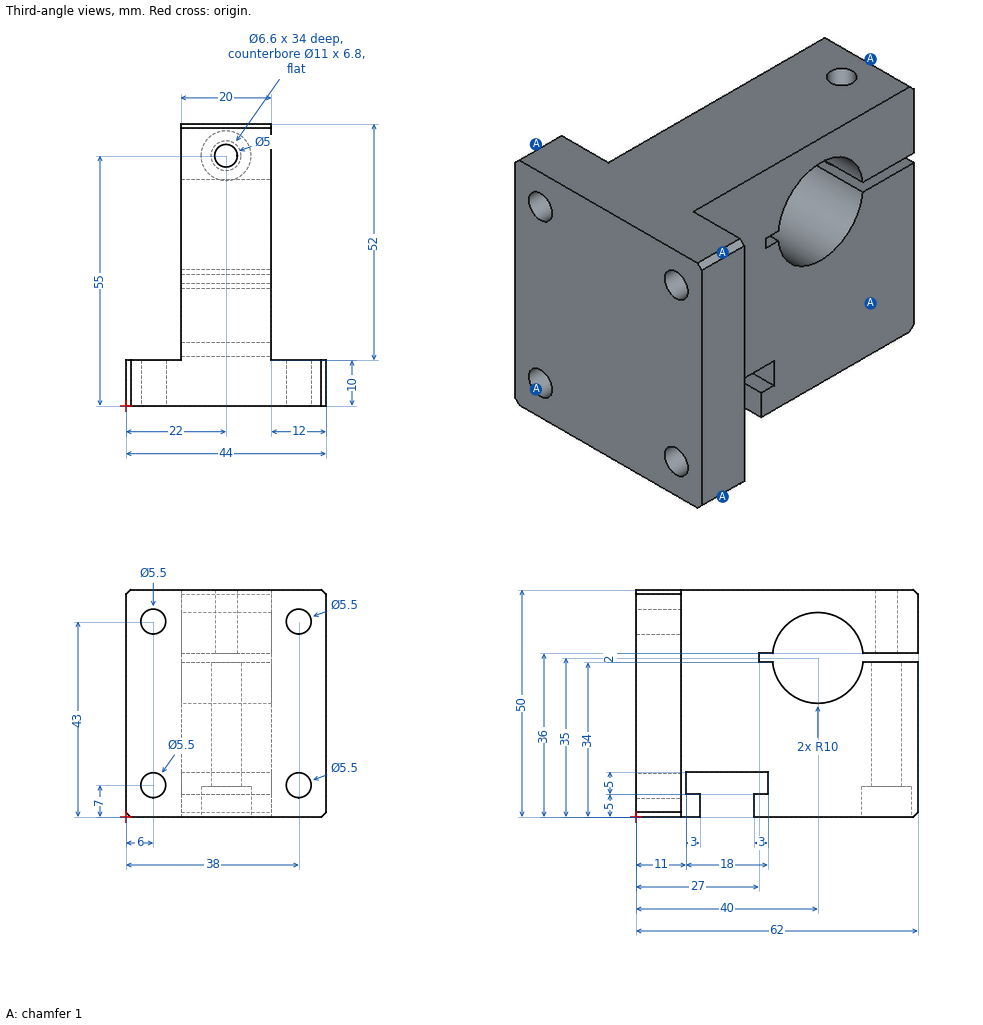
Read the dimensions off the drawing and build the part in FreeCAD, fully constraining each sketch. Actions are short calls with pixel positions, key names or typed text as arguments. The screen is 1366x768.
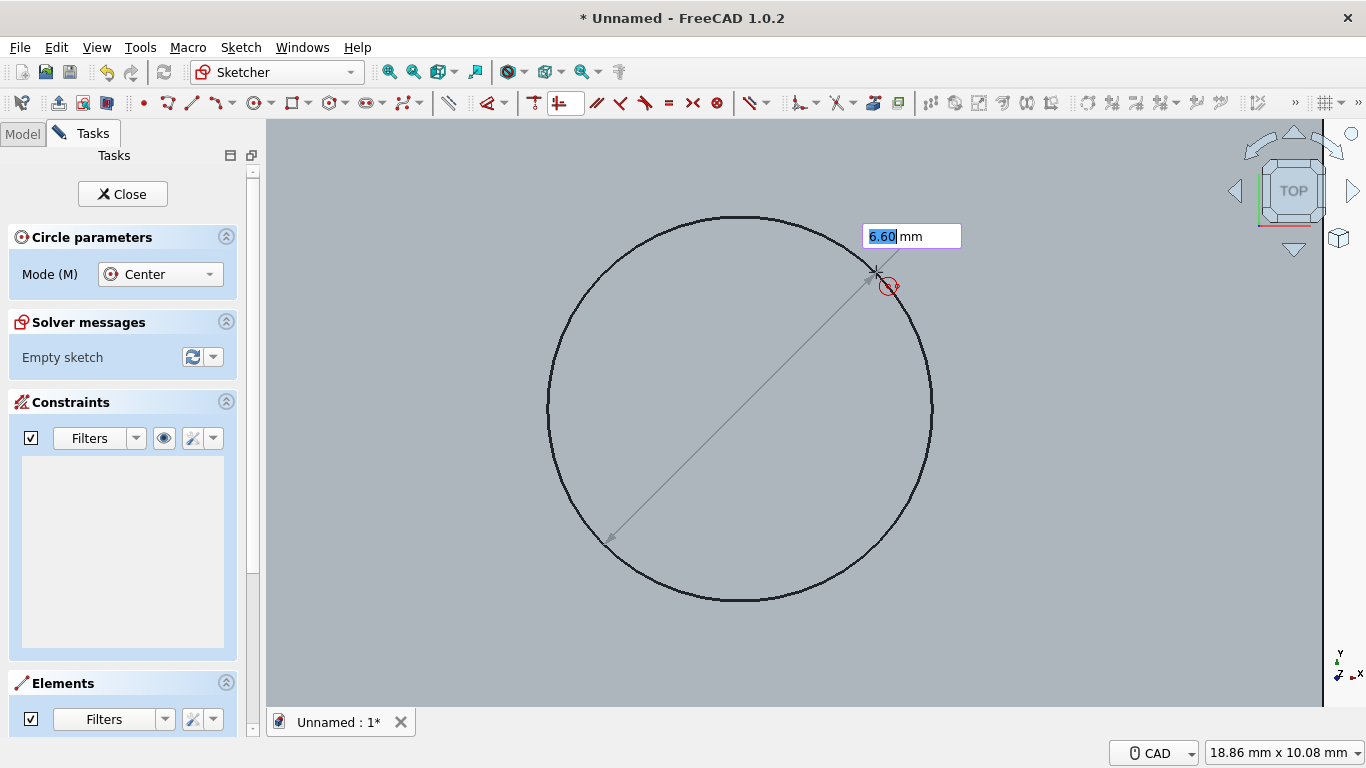
text(6.6)
key(Return)
key(Escape)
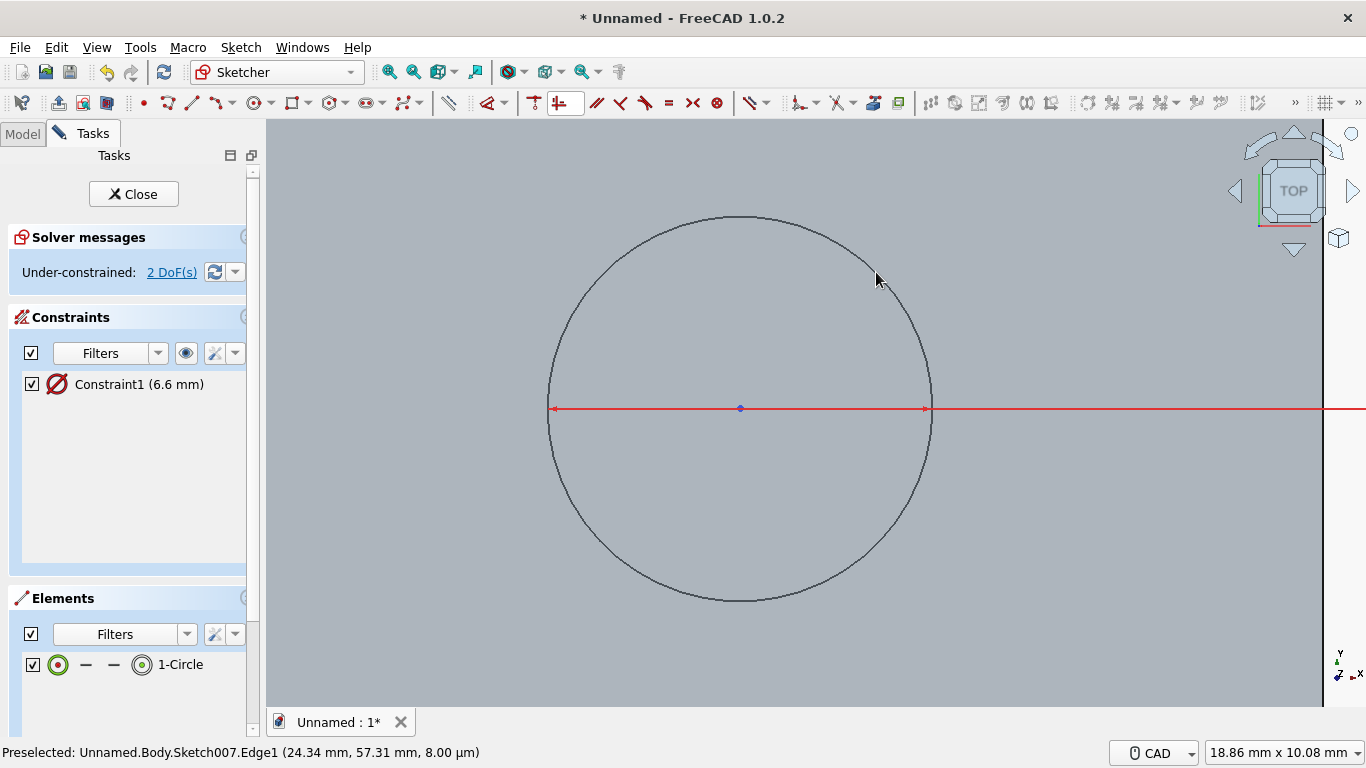
click(488, 104)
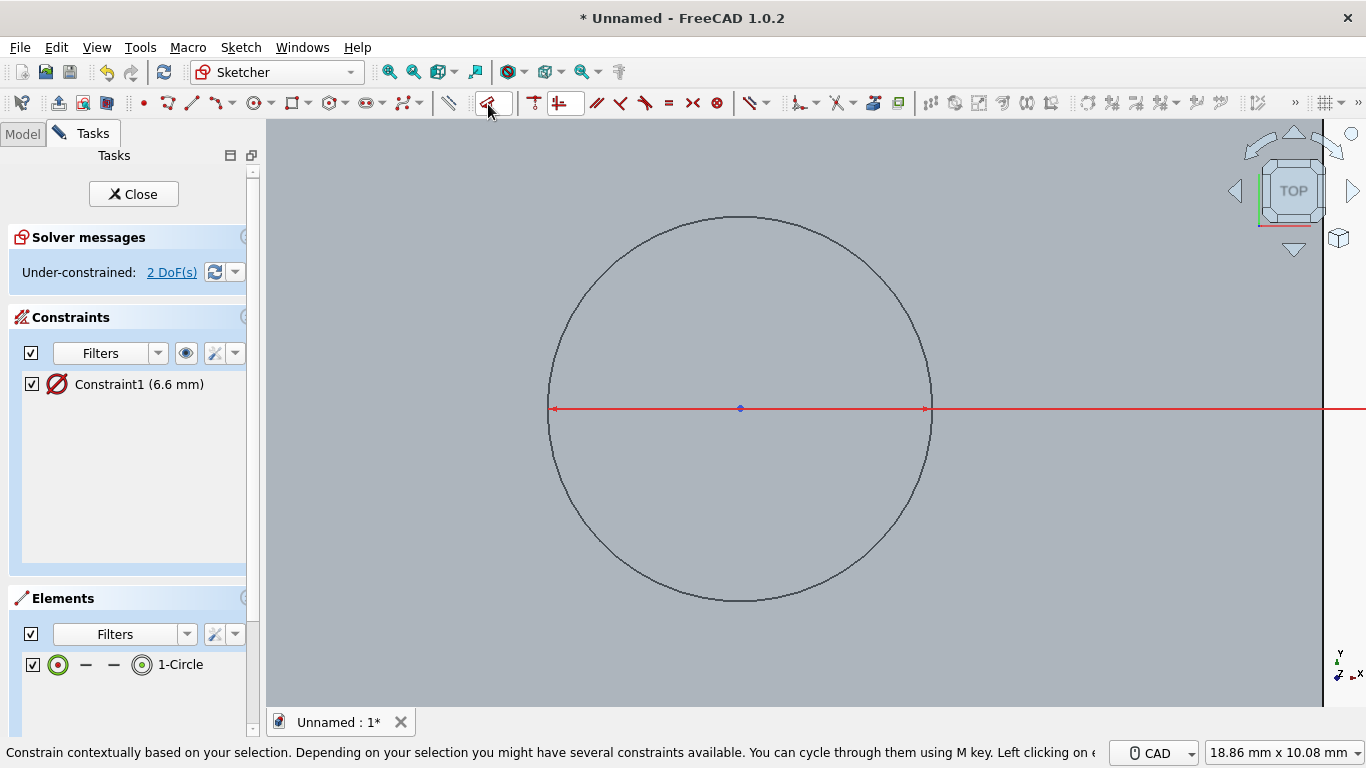
click(740, 409)
click(517, 375)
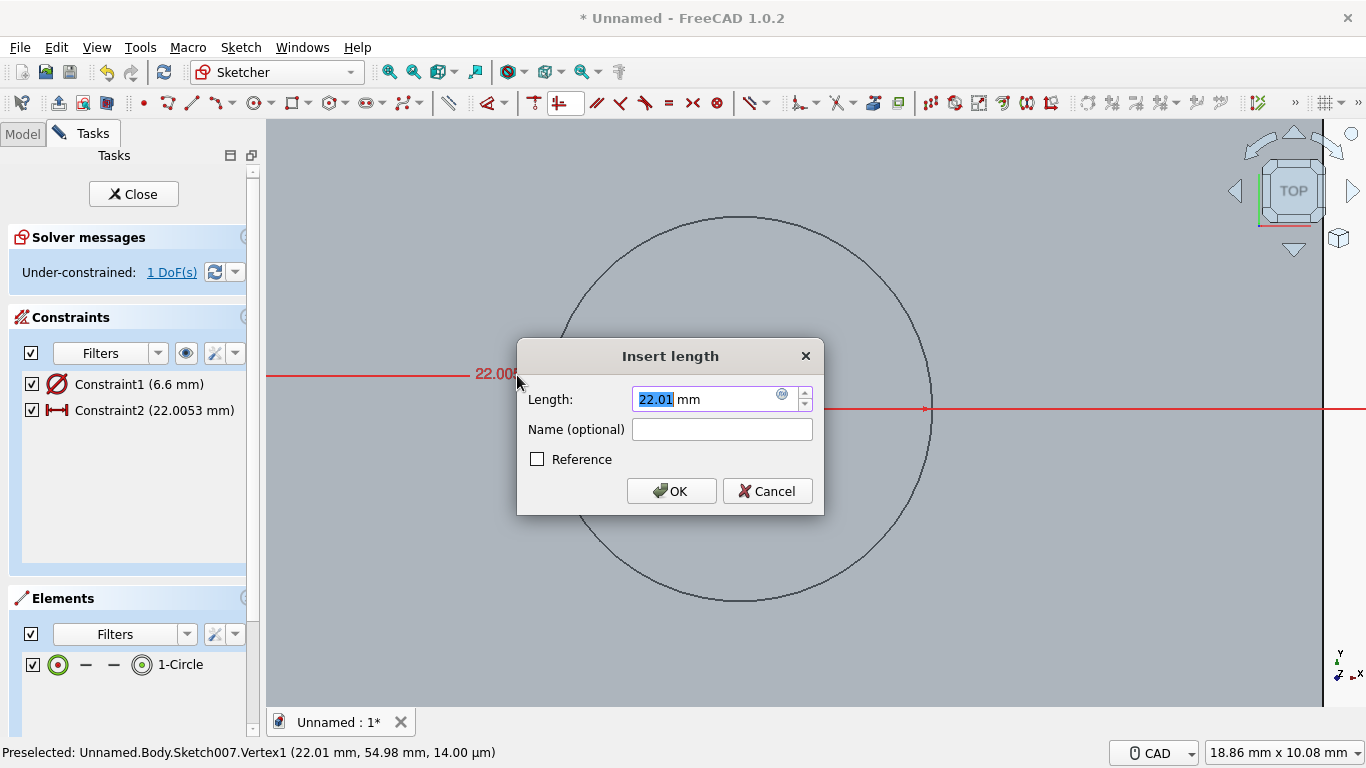
text(22)
key(Return)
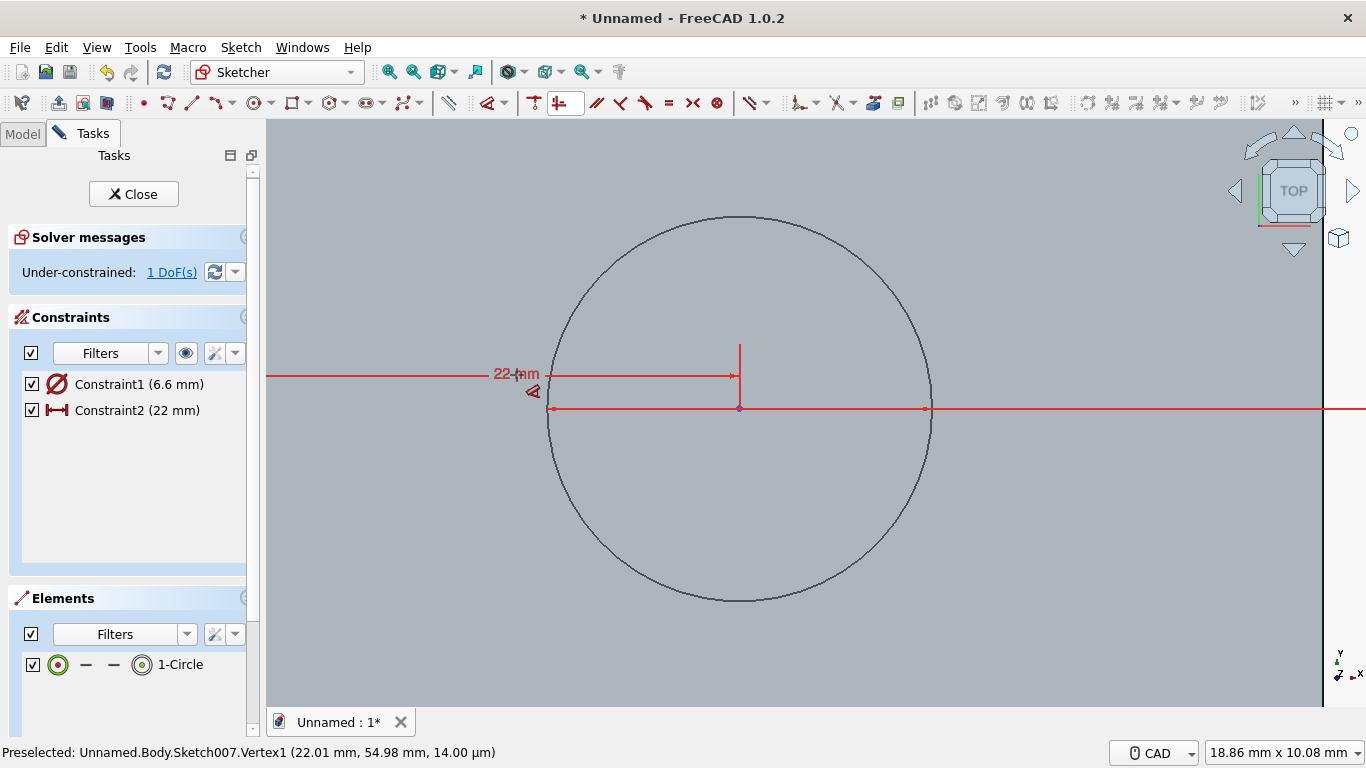
click(740, 409)
click(774, 544)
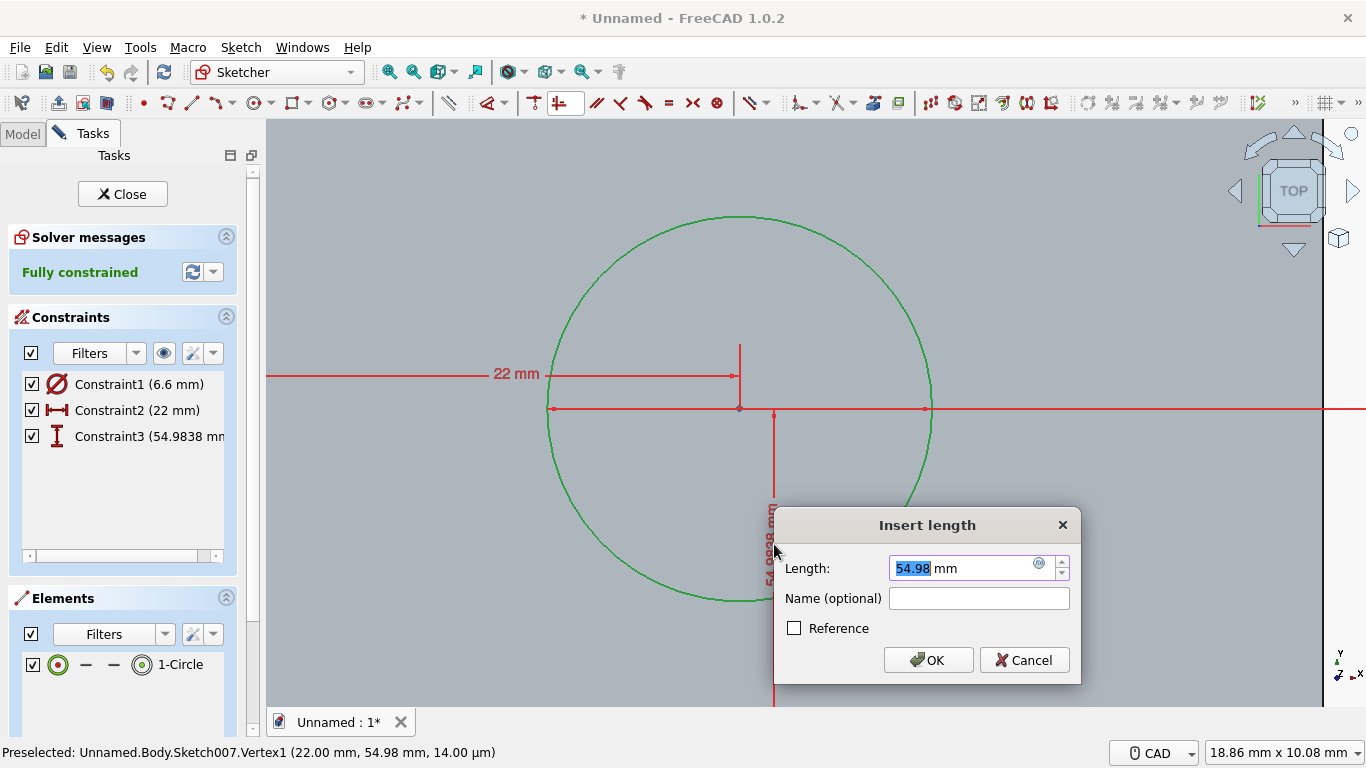
text(55)
key(Return)
key(Escape)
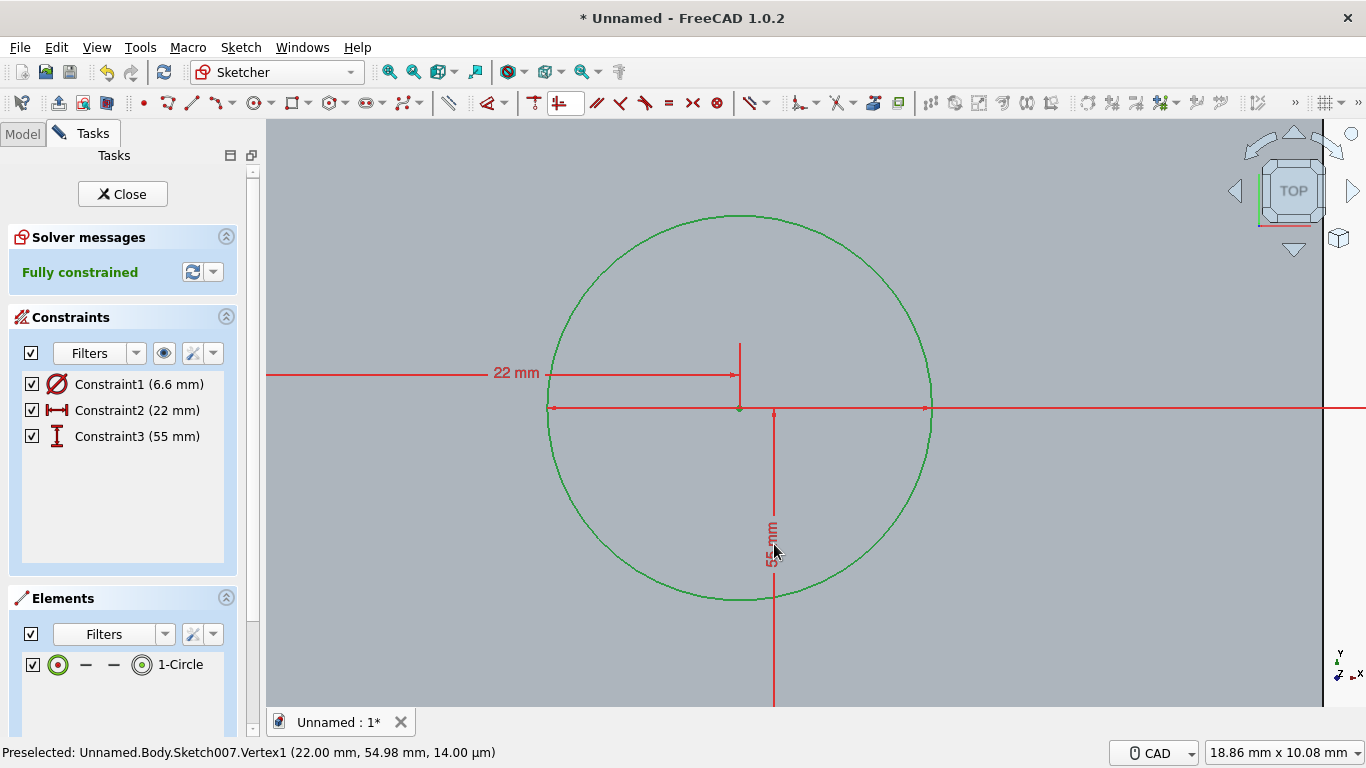
click(123, 194)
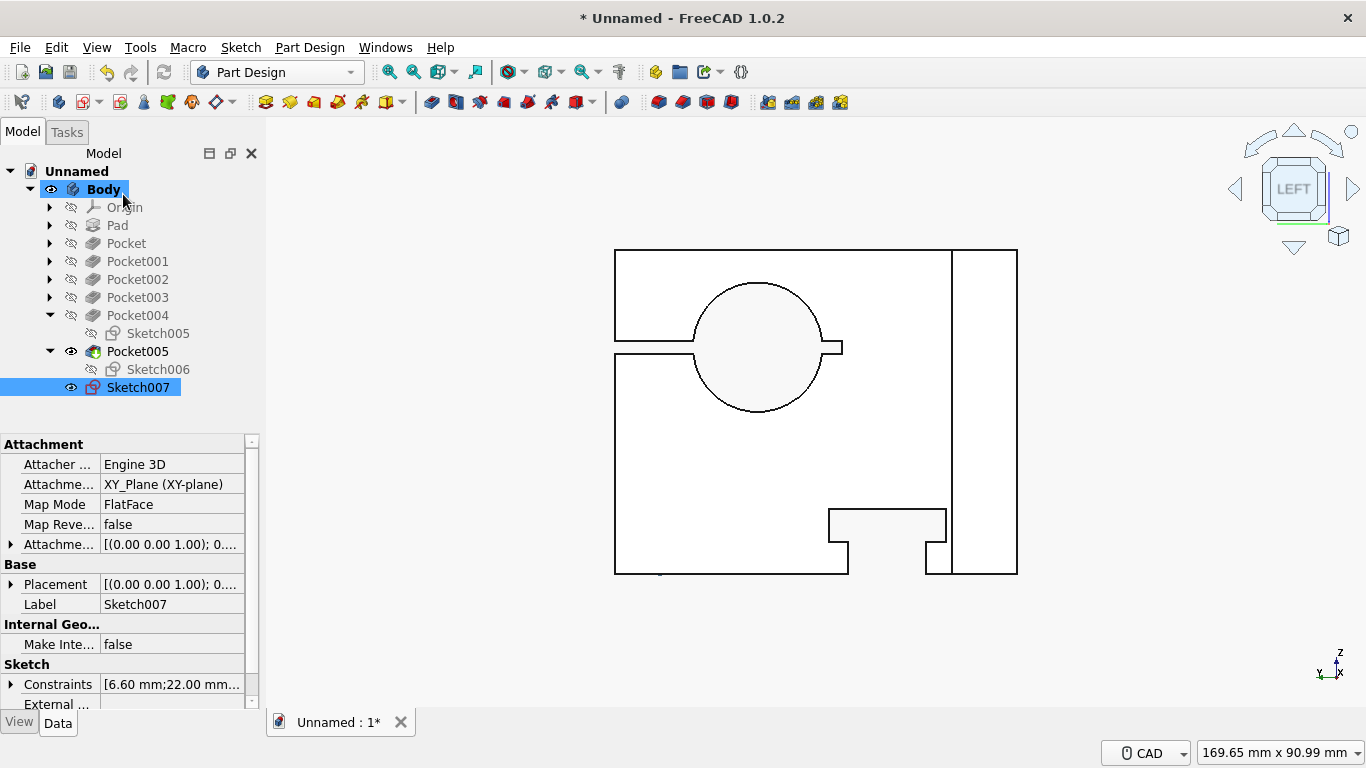
click(456, 102)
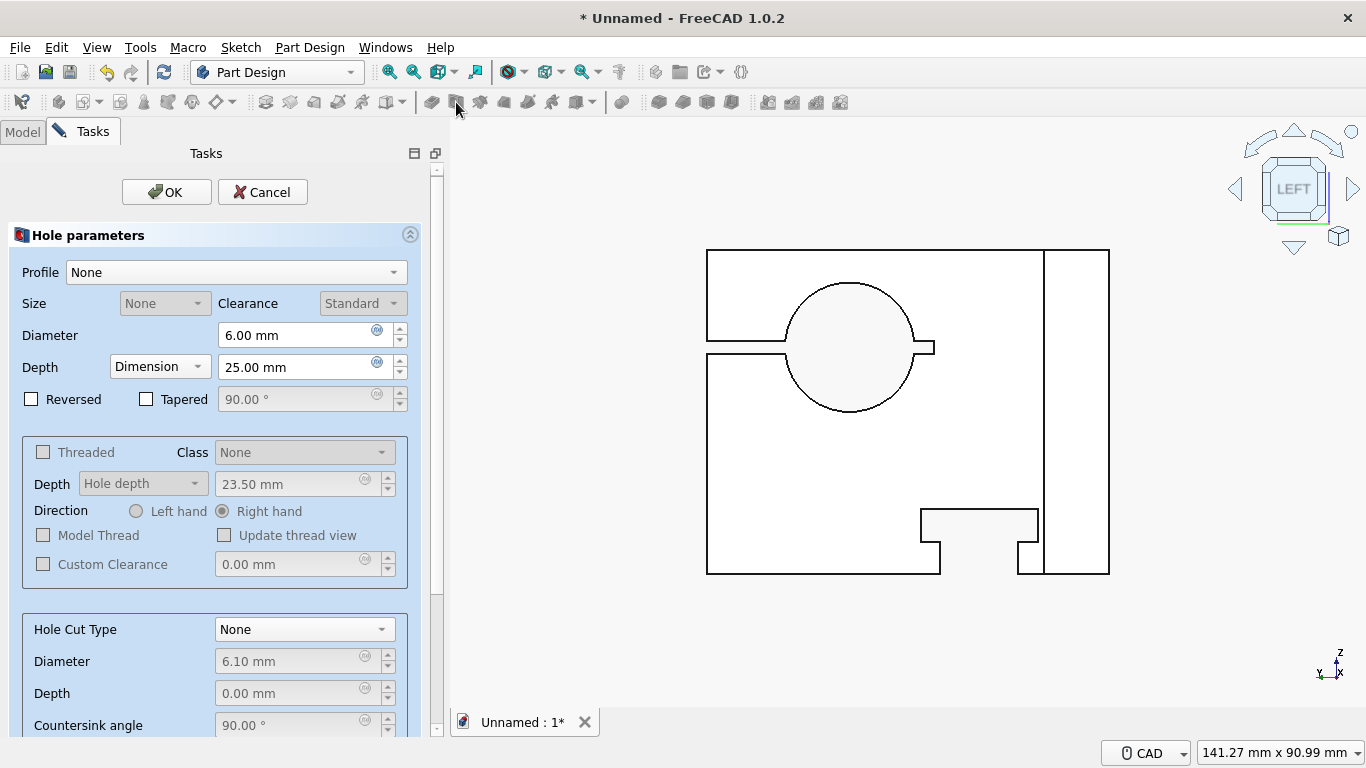
triple_click(305, 335)